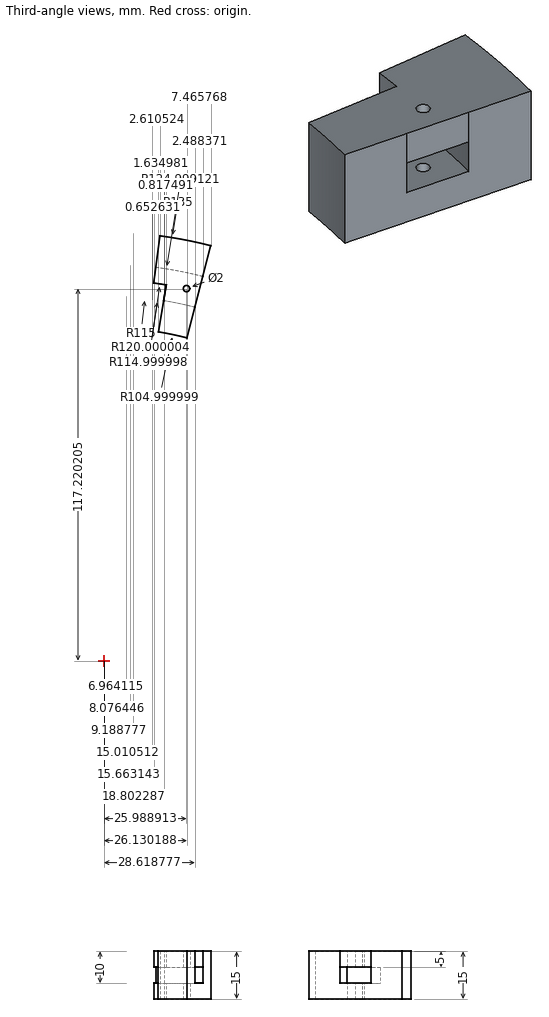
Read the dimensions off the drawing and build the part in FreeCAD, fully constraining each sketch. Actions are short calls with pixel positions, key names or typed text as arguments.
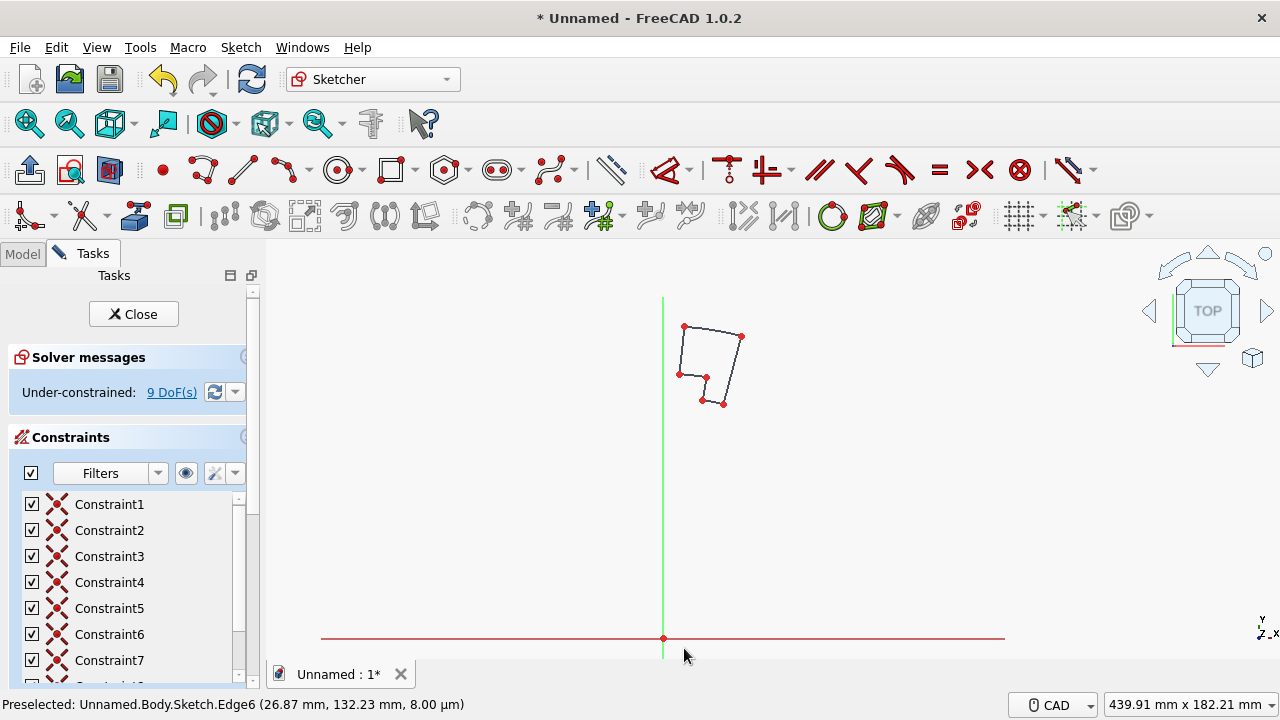
click(666, 170)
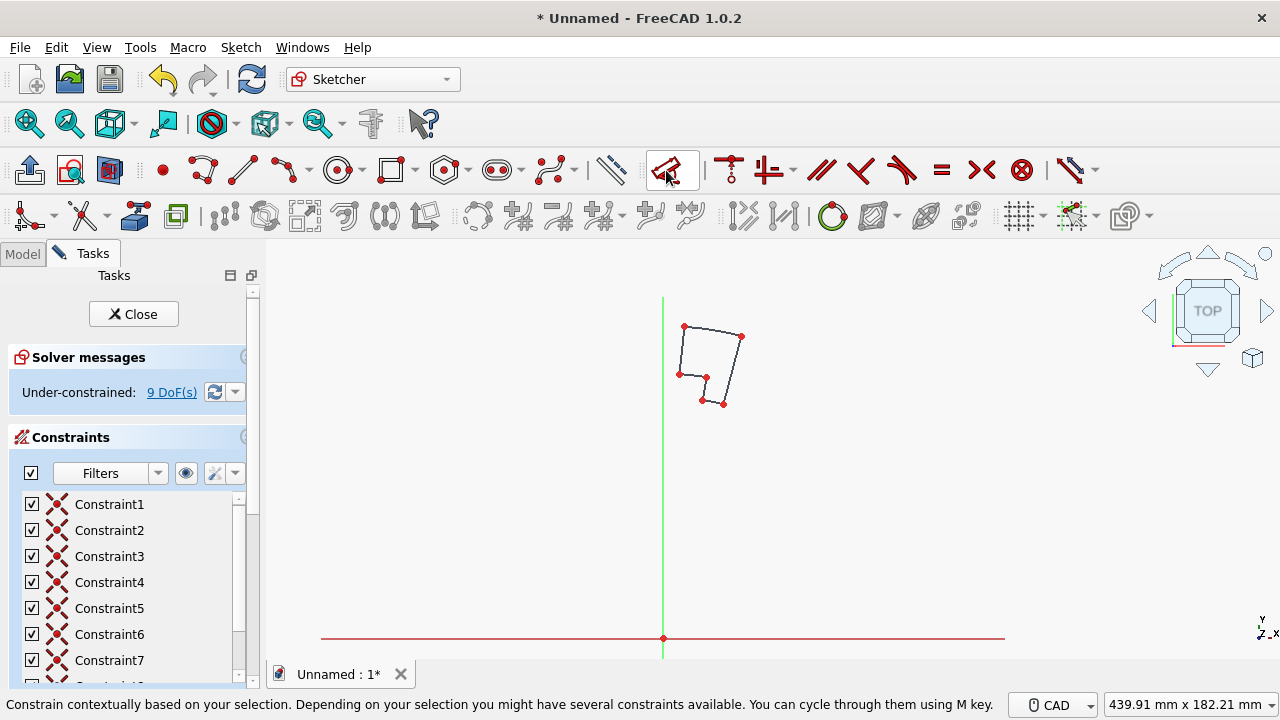
click(693, 375)
click(697, 343)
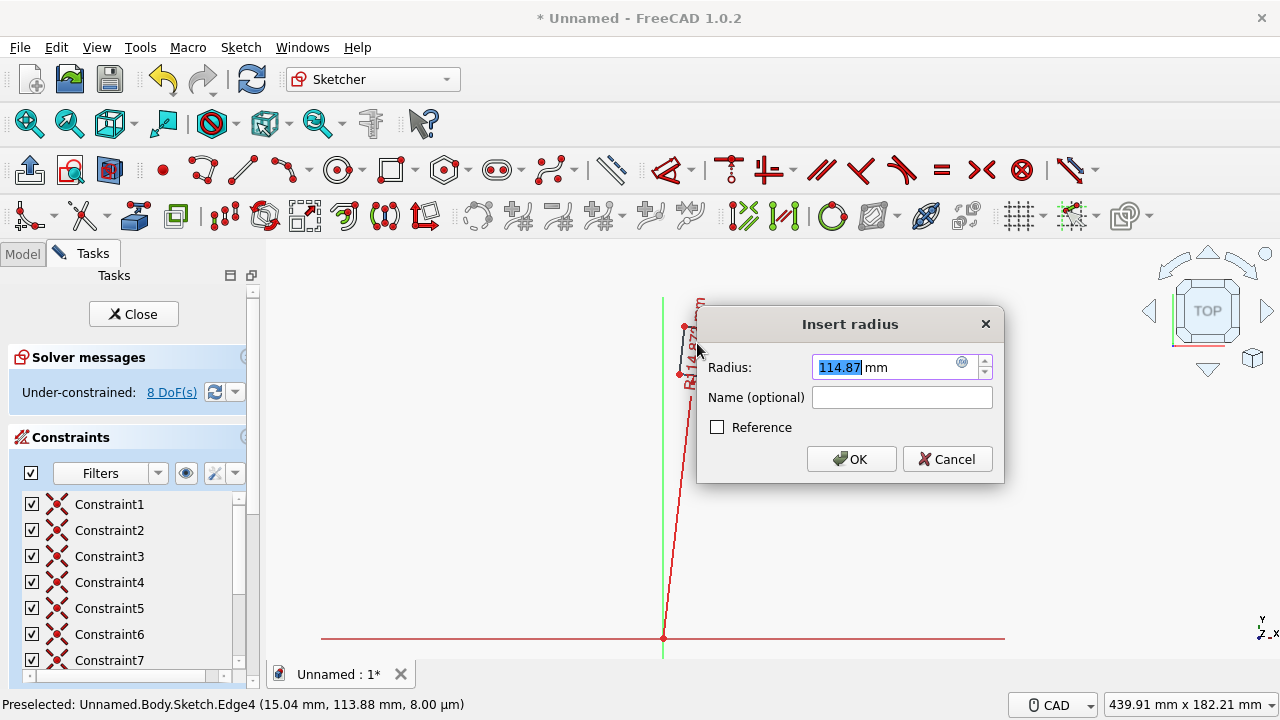
text(115)
key(Return)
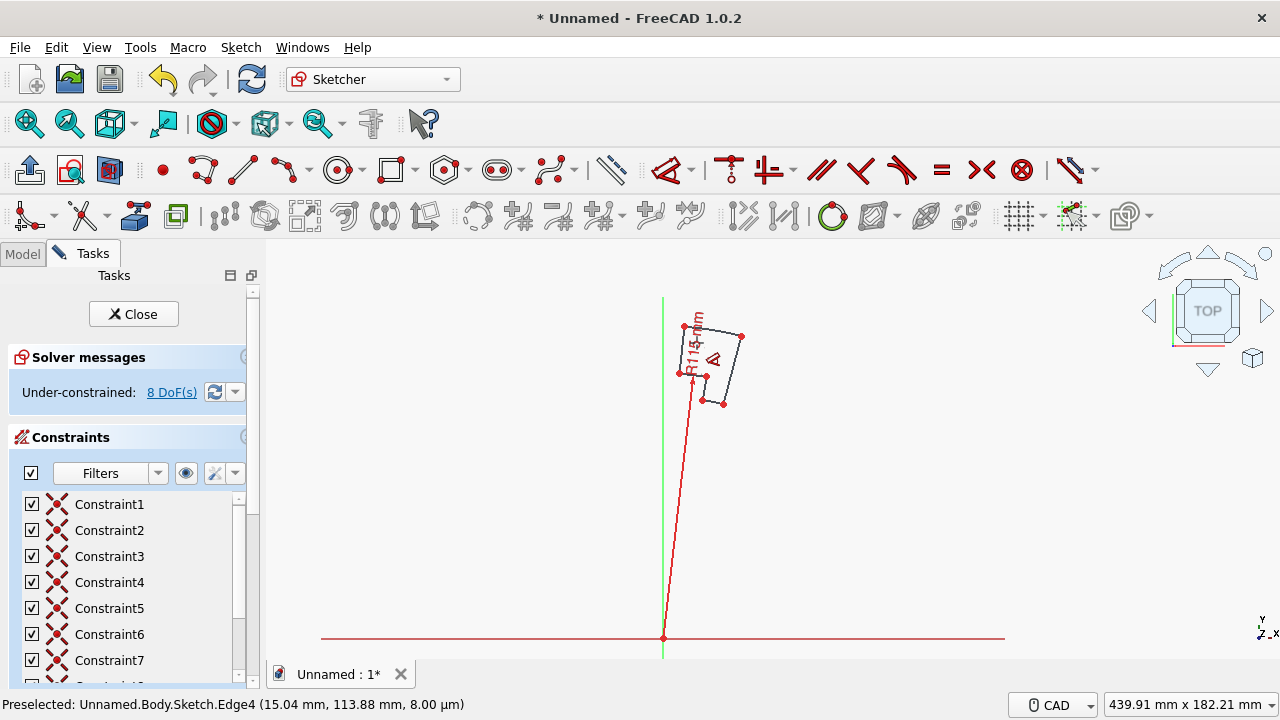
scroll(713, 402, up, 2)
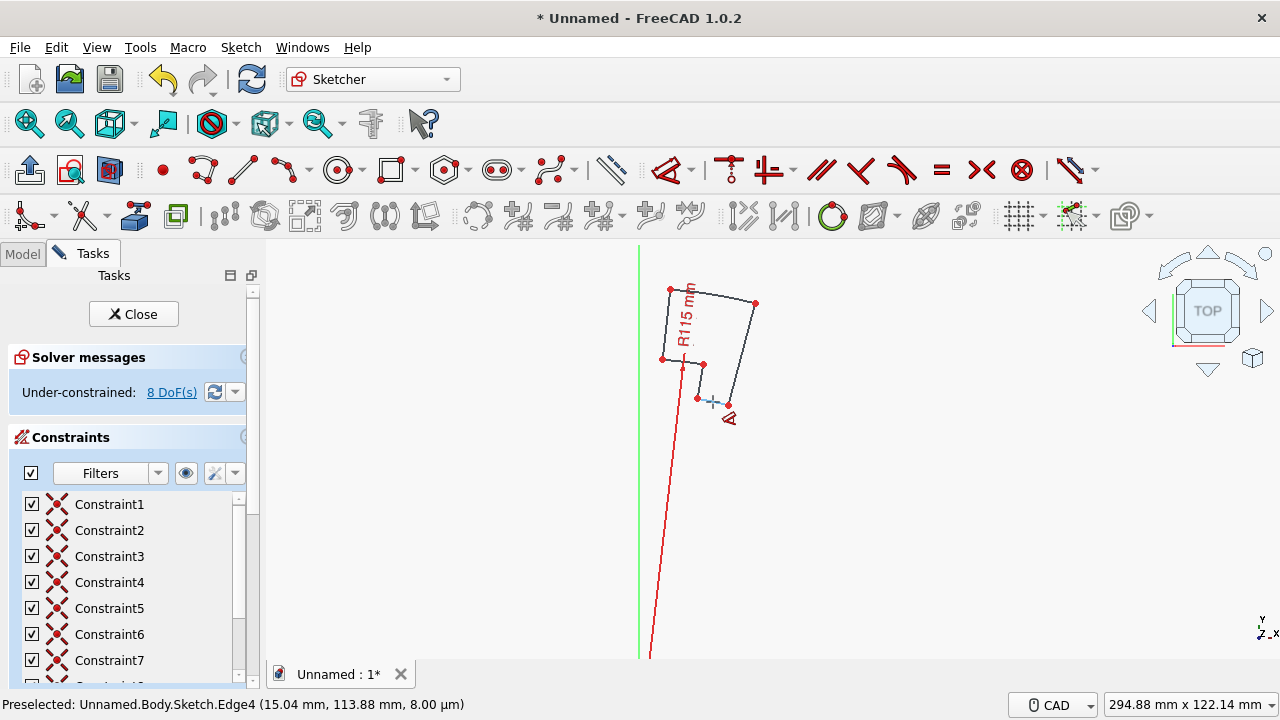
click(713, 402)
click(720, 371)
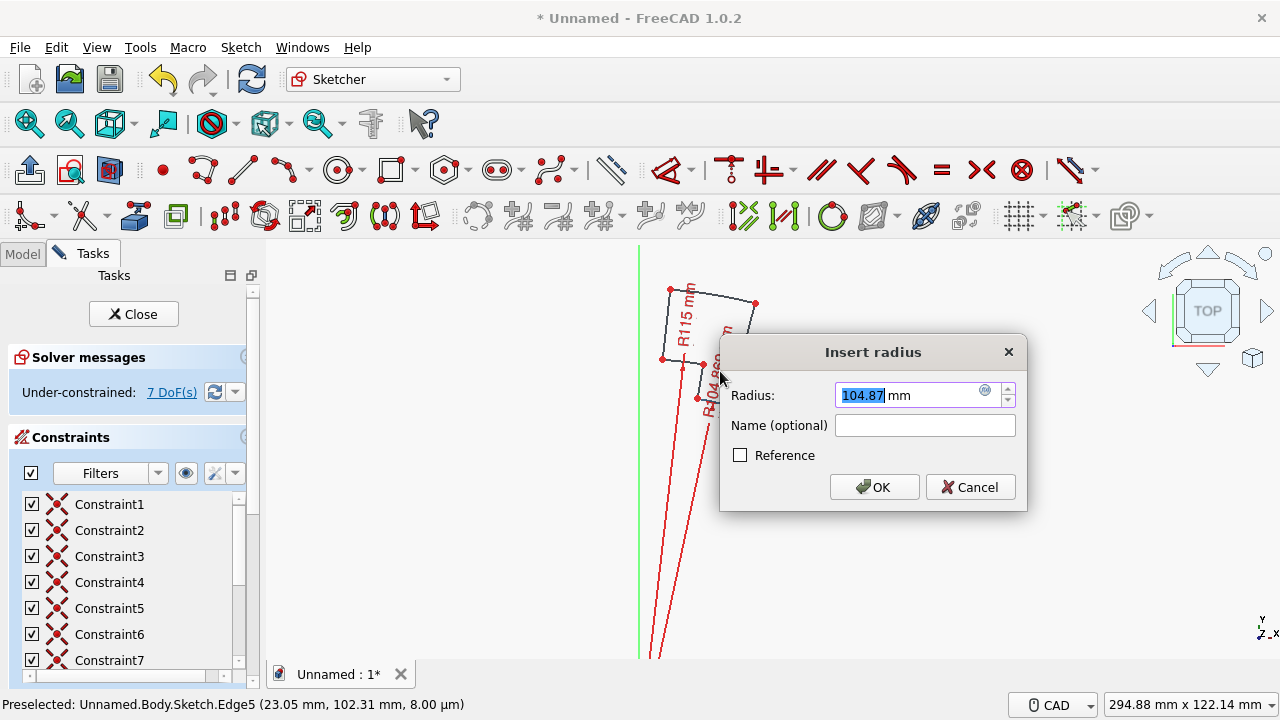
text(104.999999)
key(Return)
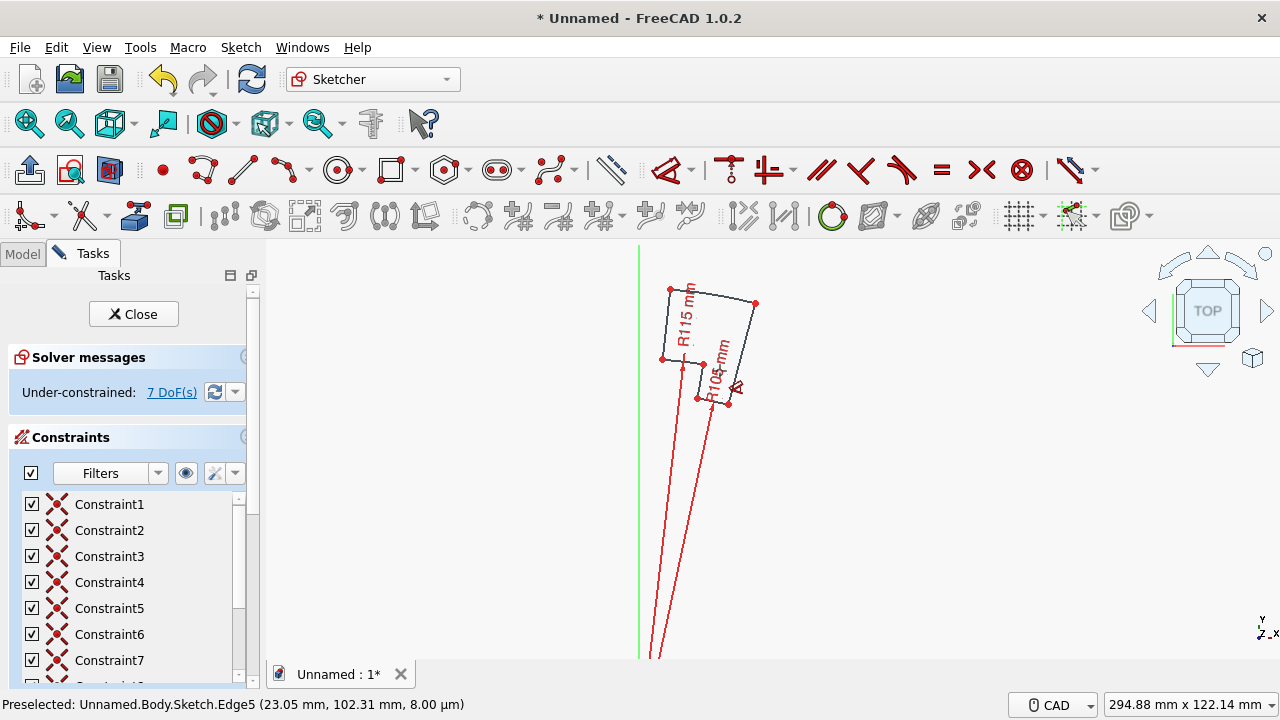
click(730, 298)
click(958, 373)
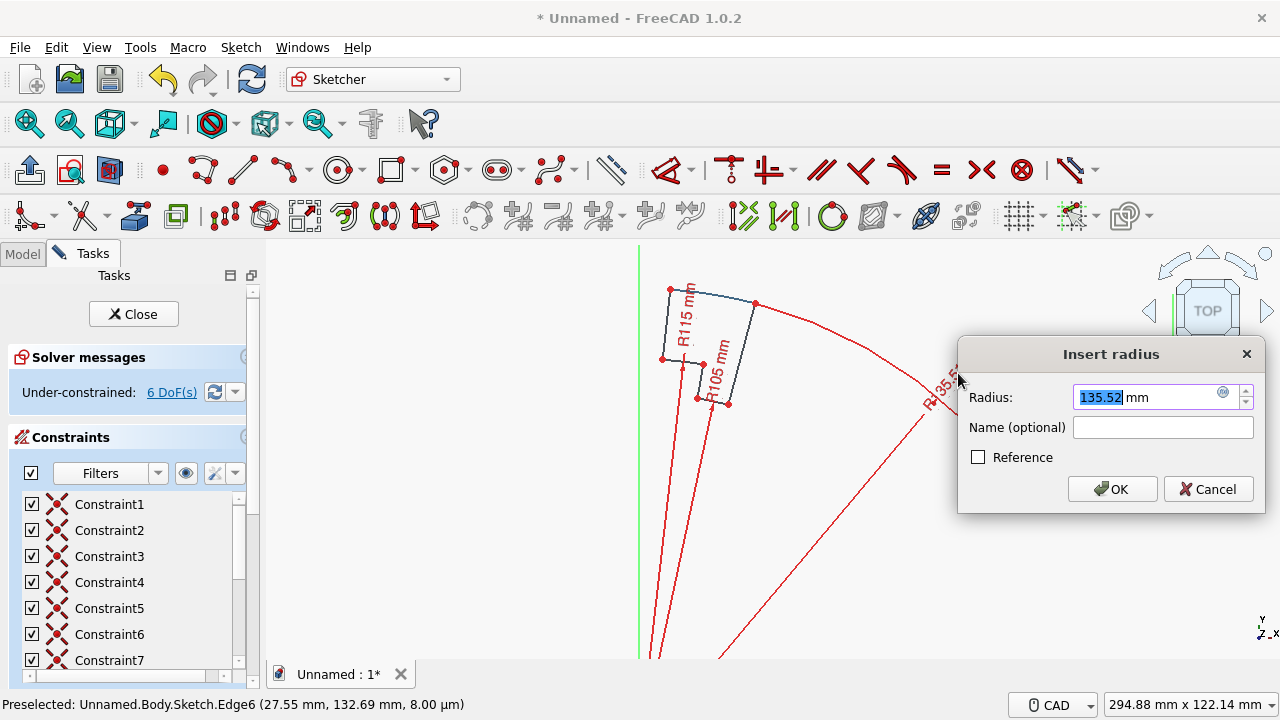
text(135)
key(Return)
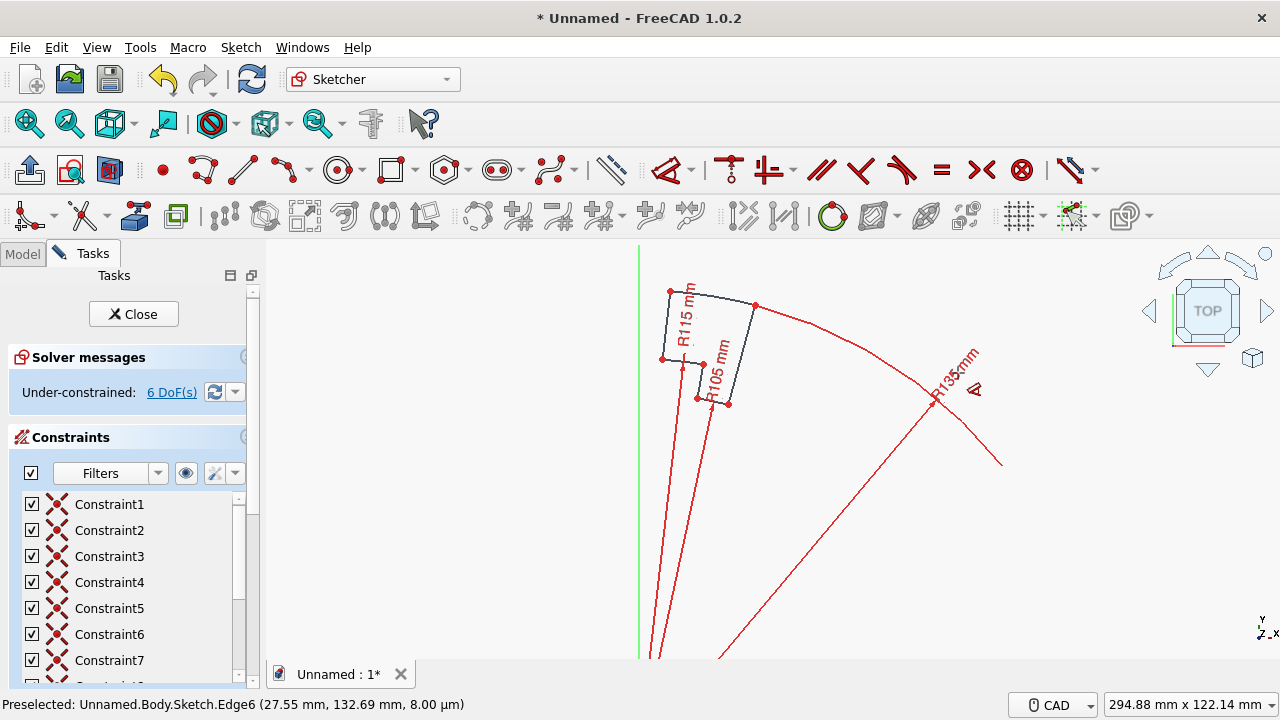
scroll(670, 291, up, 2)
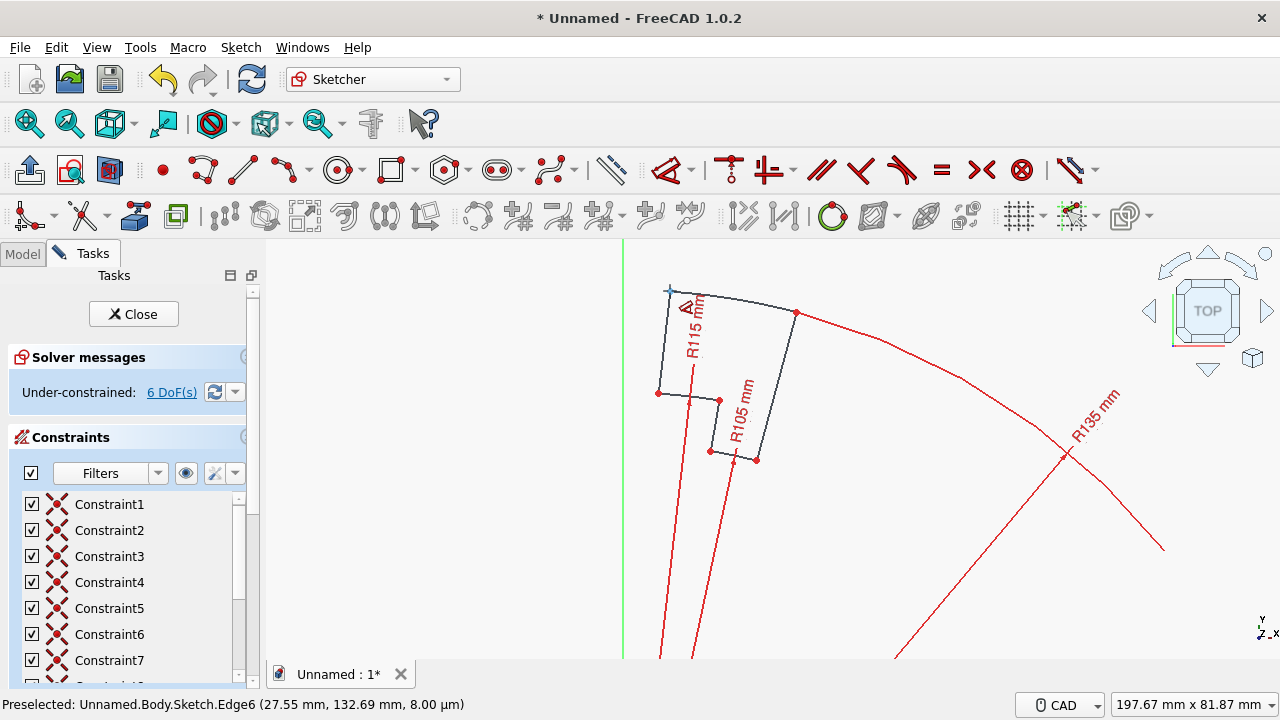
click(670, 292)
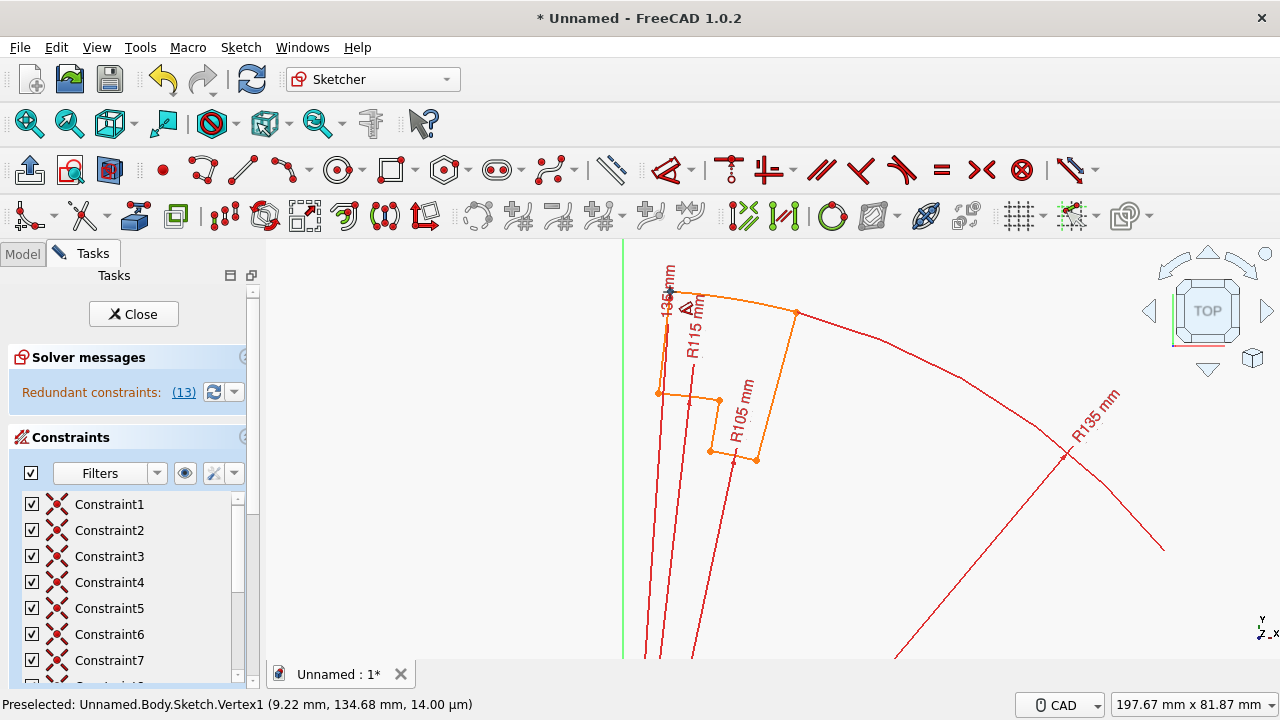
key(Escape)
key(Escape)